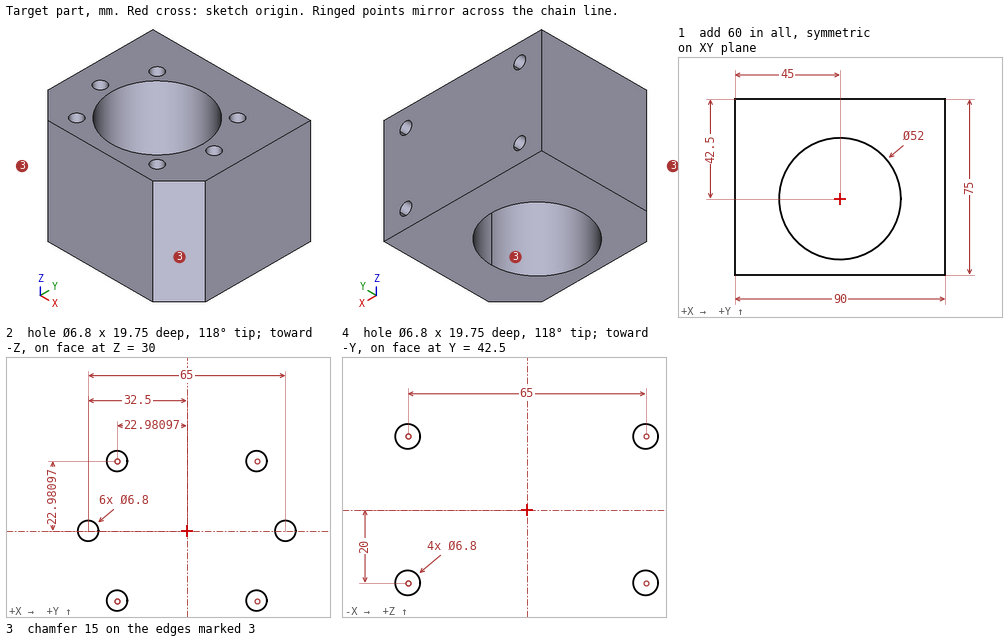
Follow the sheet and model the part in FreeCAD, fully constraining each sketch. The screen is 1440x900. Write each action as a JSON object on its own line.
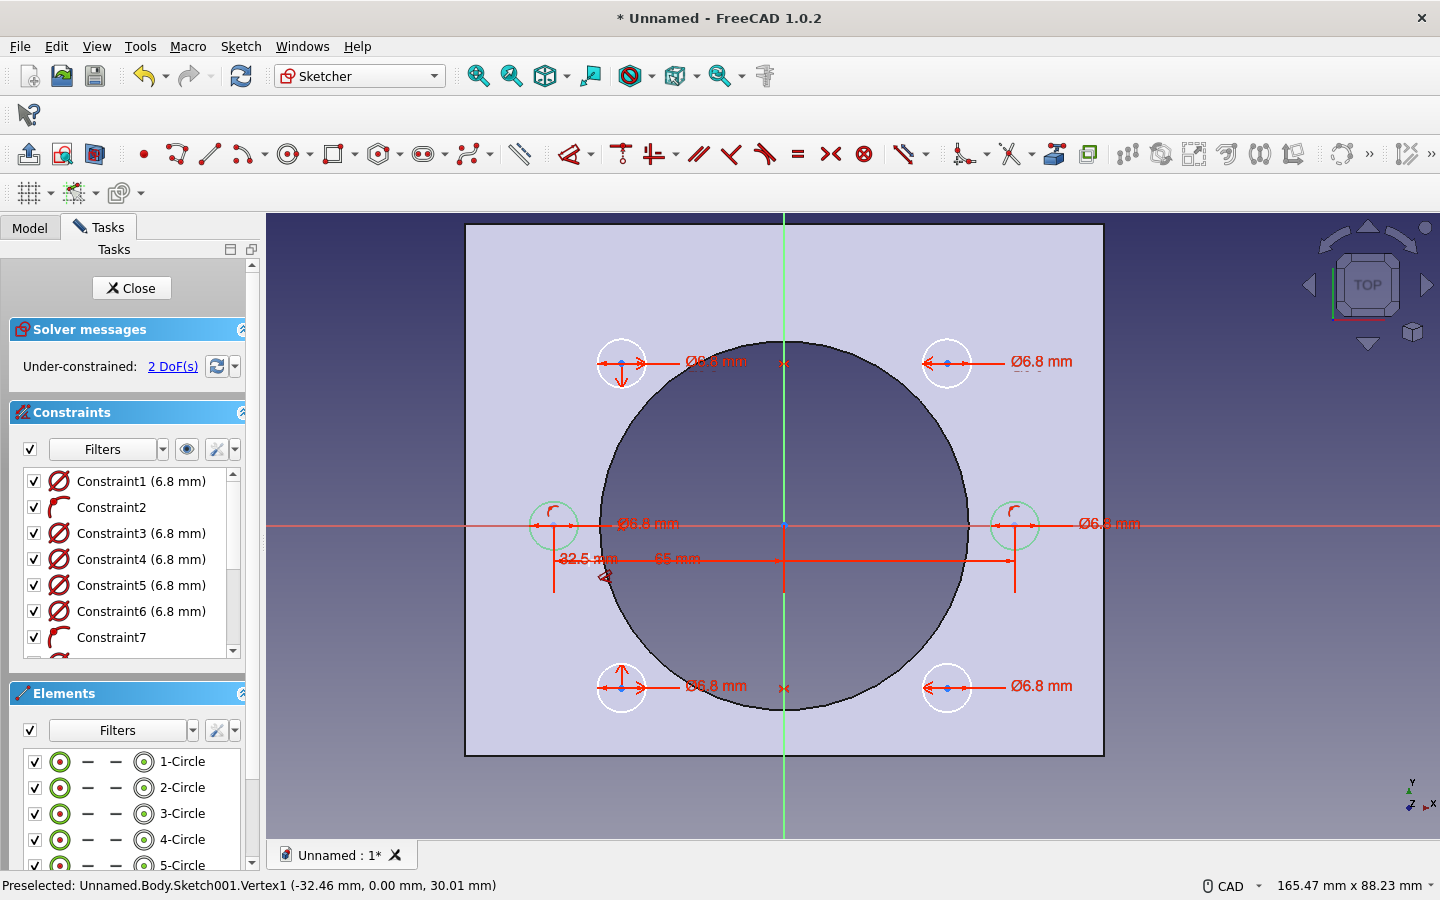
{"action": "left_click", "coordinate": [622, 363]}
{"action": "left_click", "coordinate": [703, 329]}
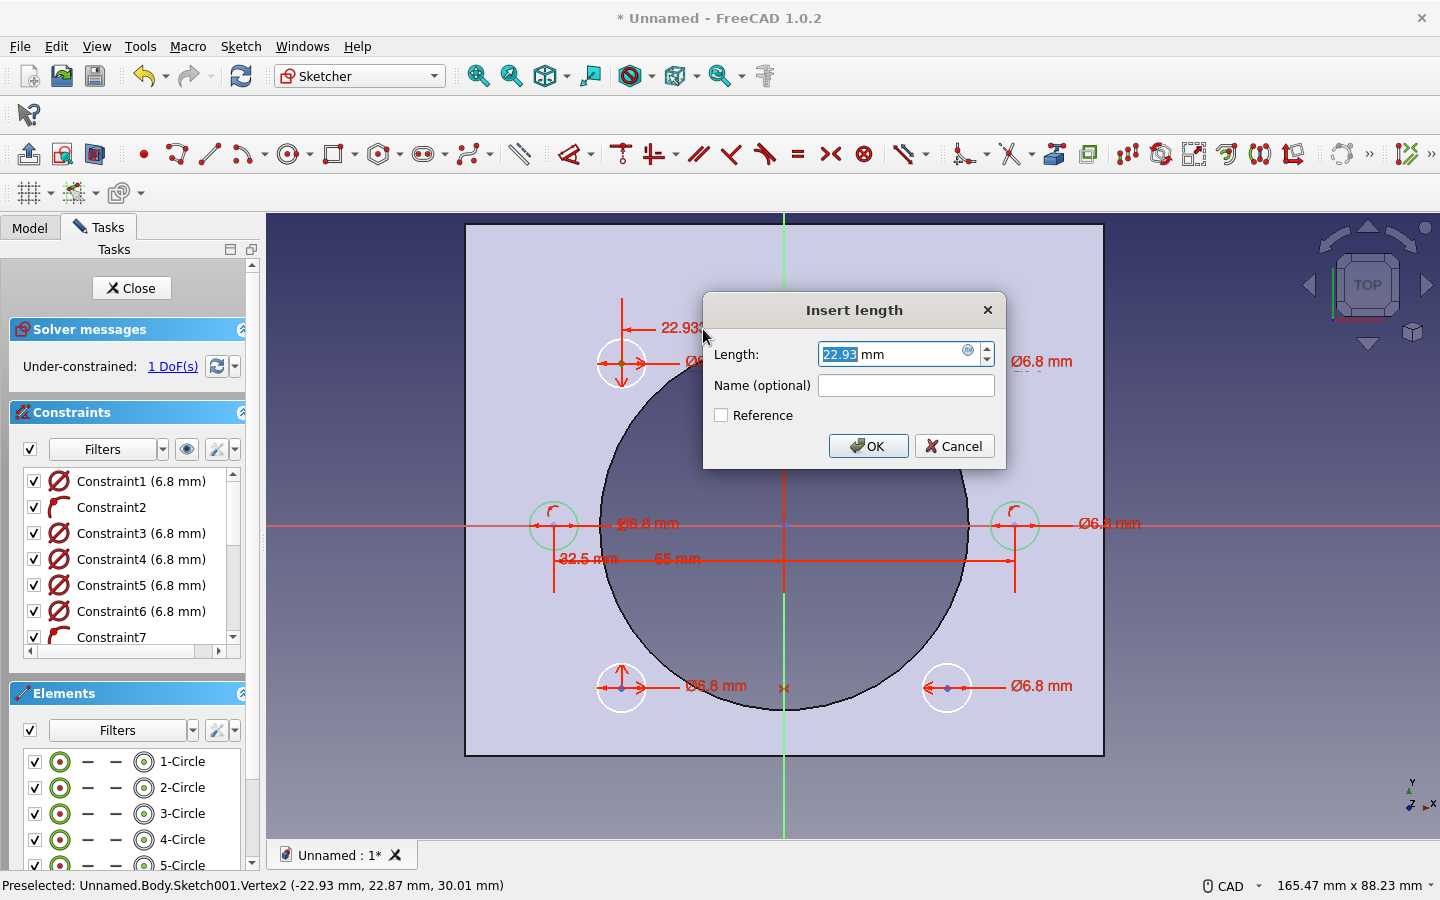
{"action": "type", "text": "22.98097"}
{"action": "key", "text": "Return"}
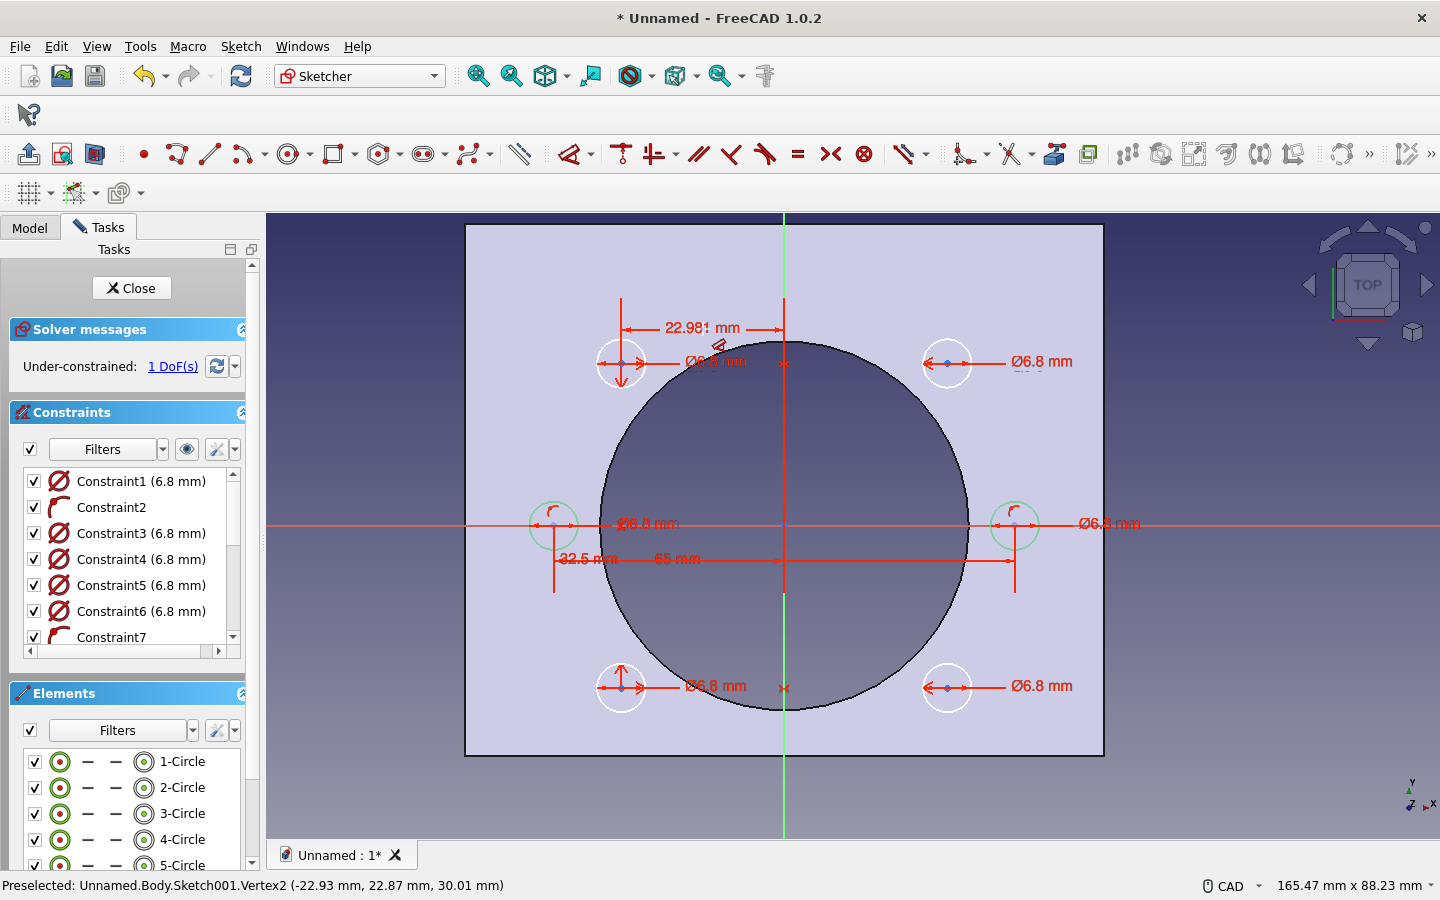
{"action": "left_click", "coordinate": [621, 363]}
{"action": "left_click", "coordinate": [587, 445]}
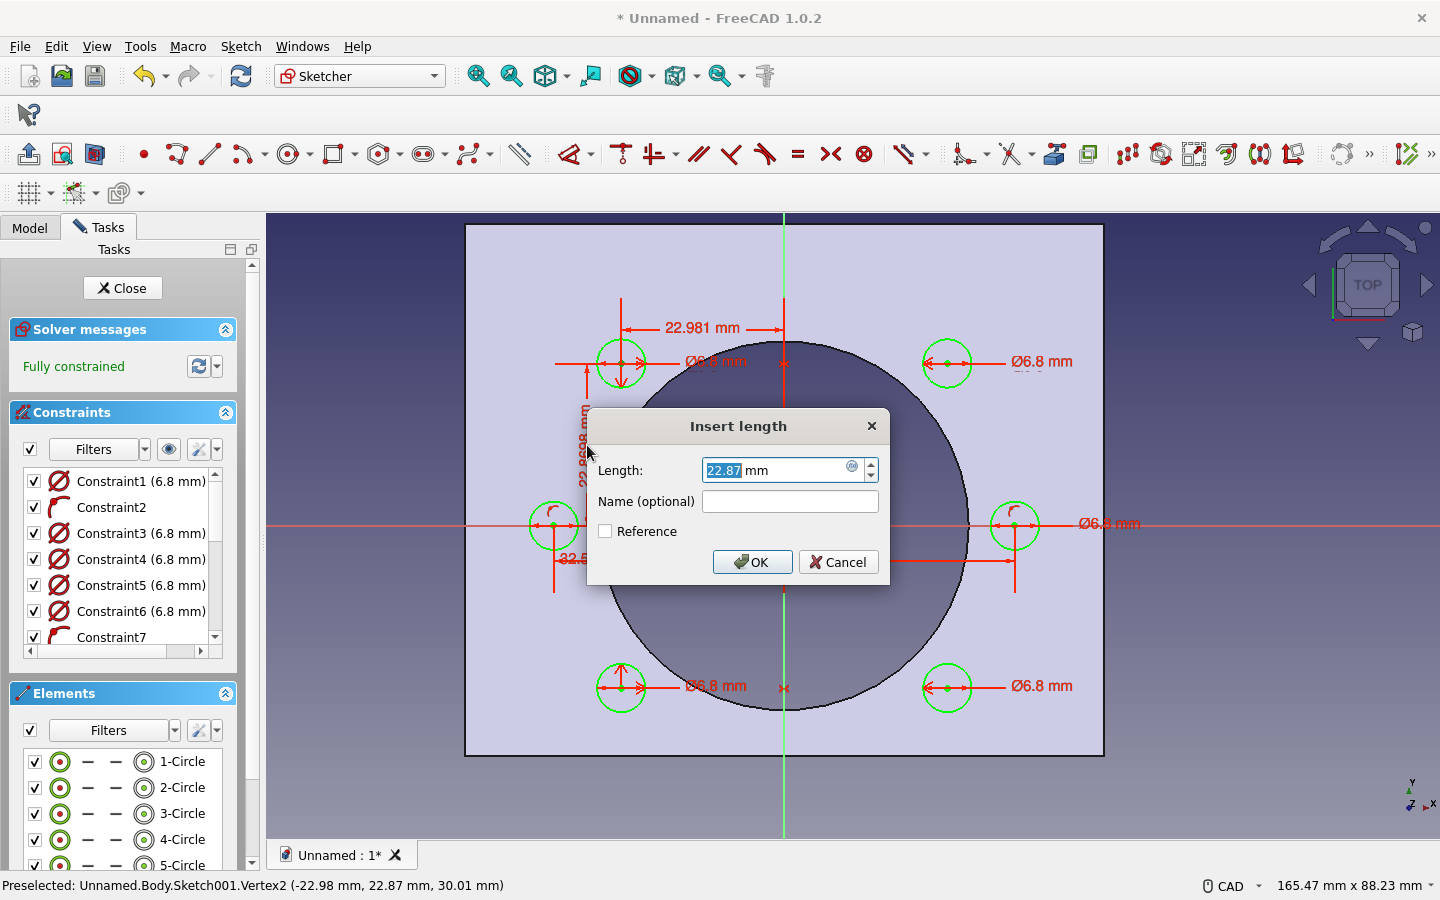
{"action": "type", "text": "22.98097"}
{"action": "key", "text": "Return"}
{"action": "key", "text": "Escape"}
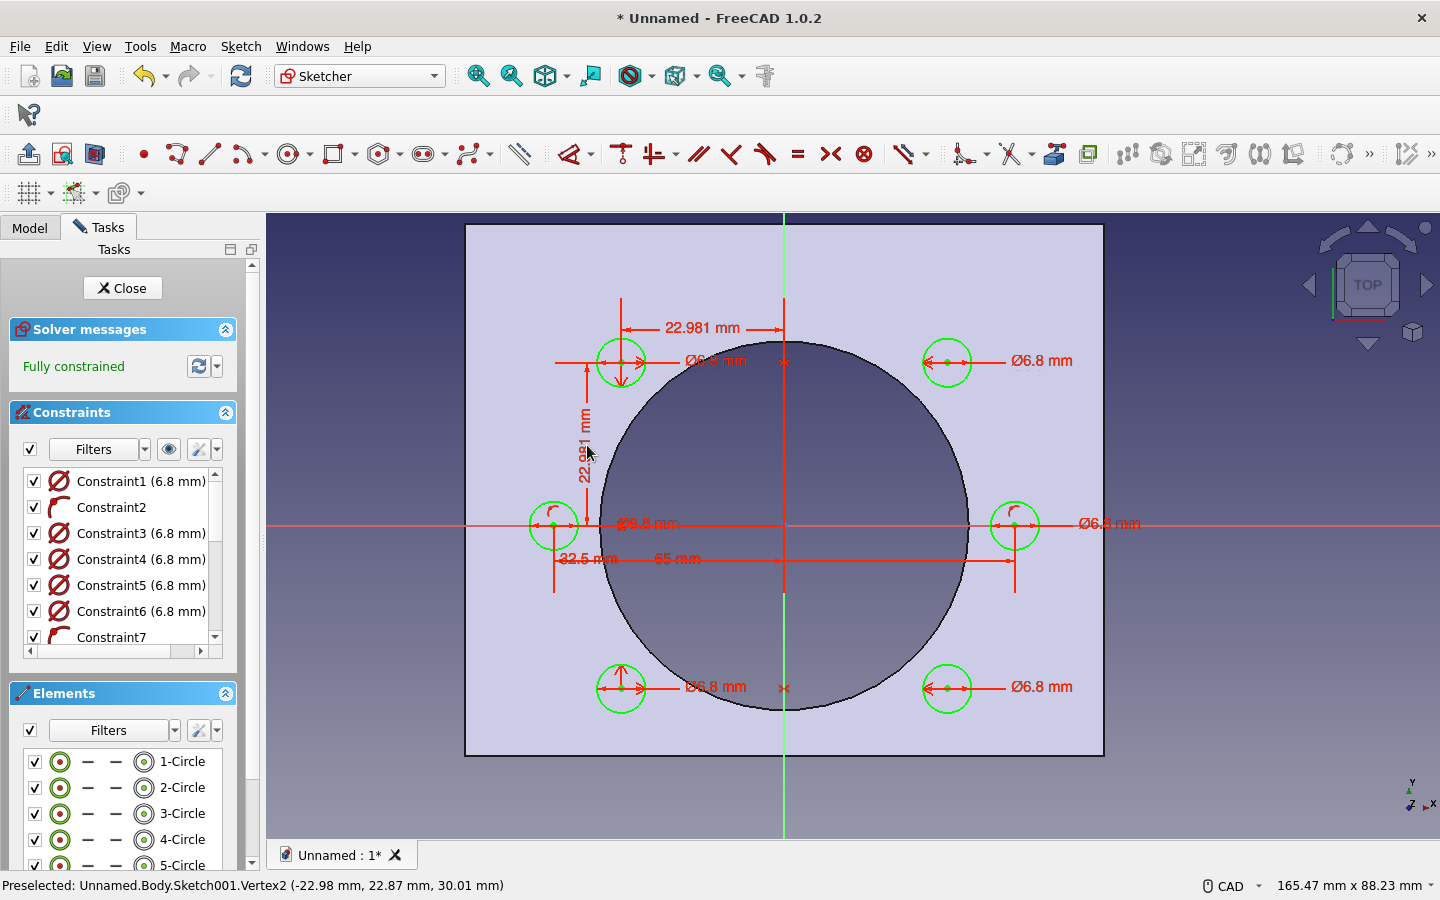
{"action": "left_click", "coordinate": [123, 288]}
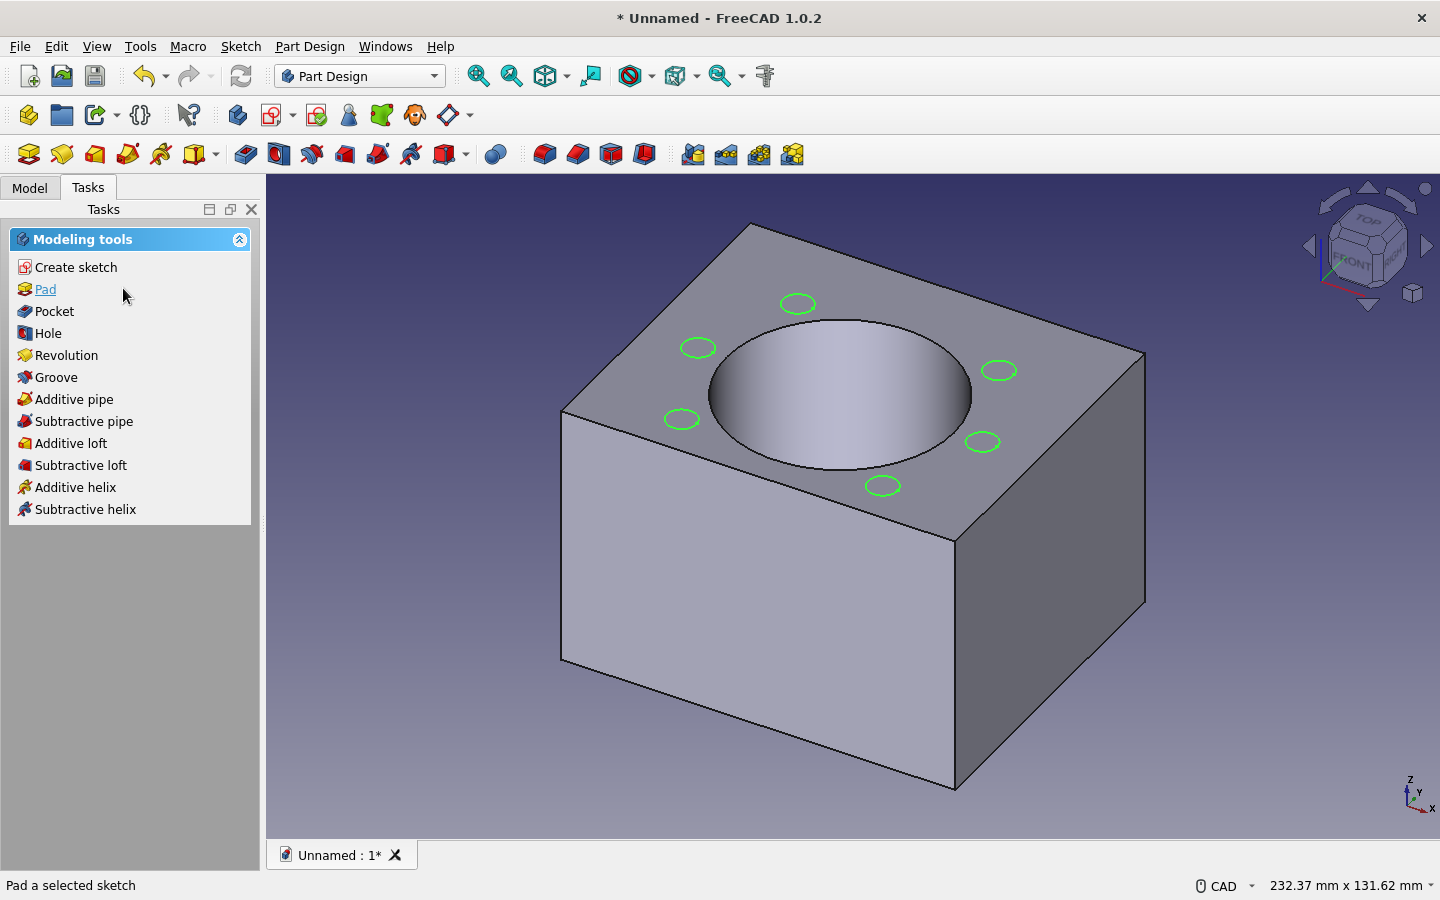
{"action": "left_click", "coordinate": [279, 154]}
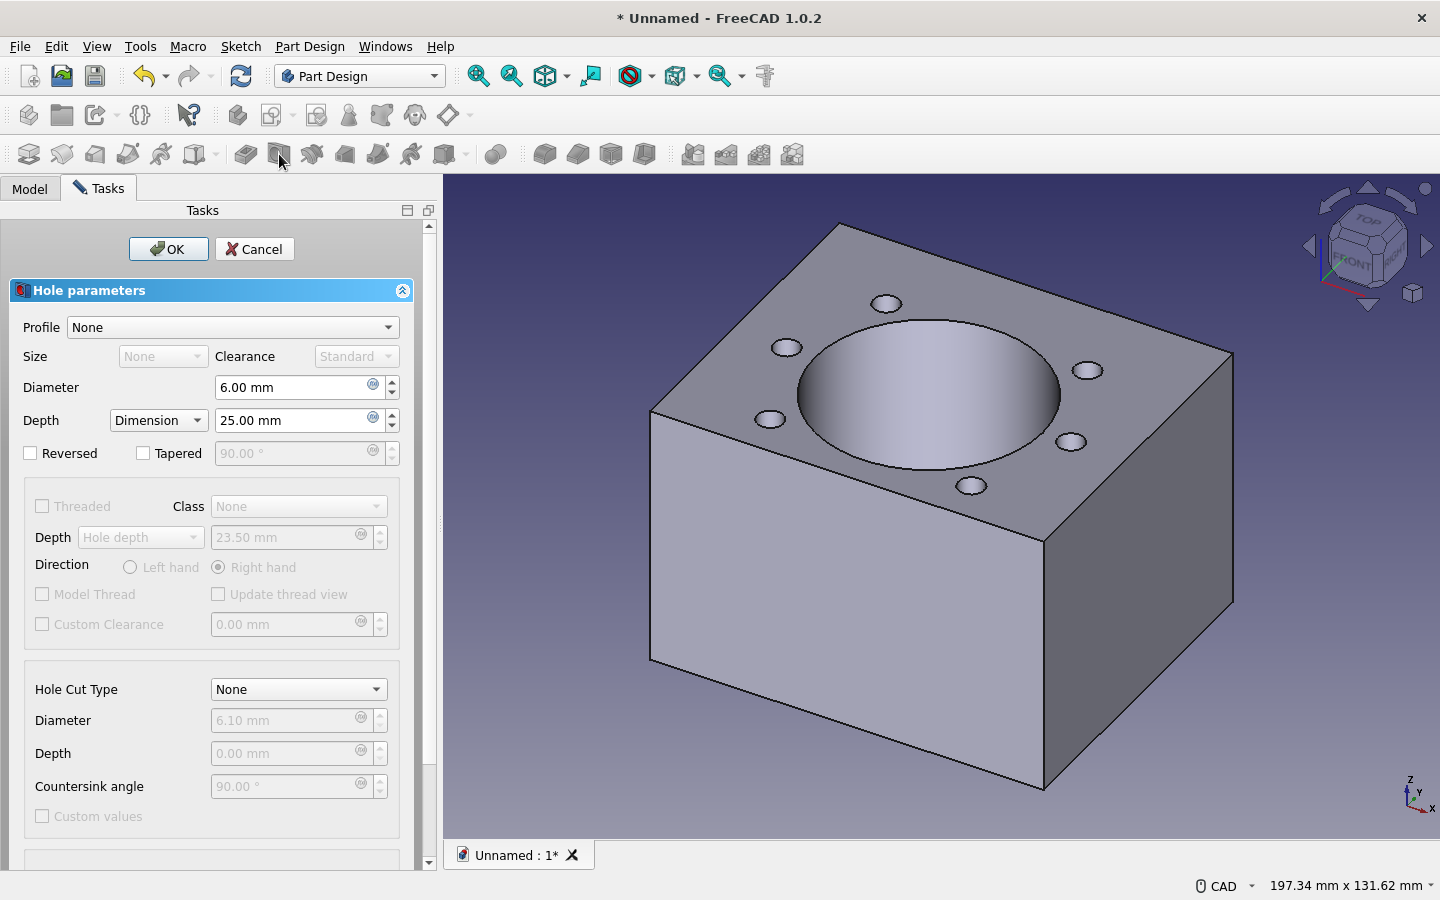
{"action": "triple_click", "coordinate": [300, 388]}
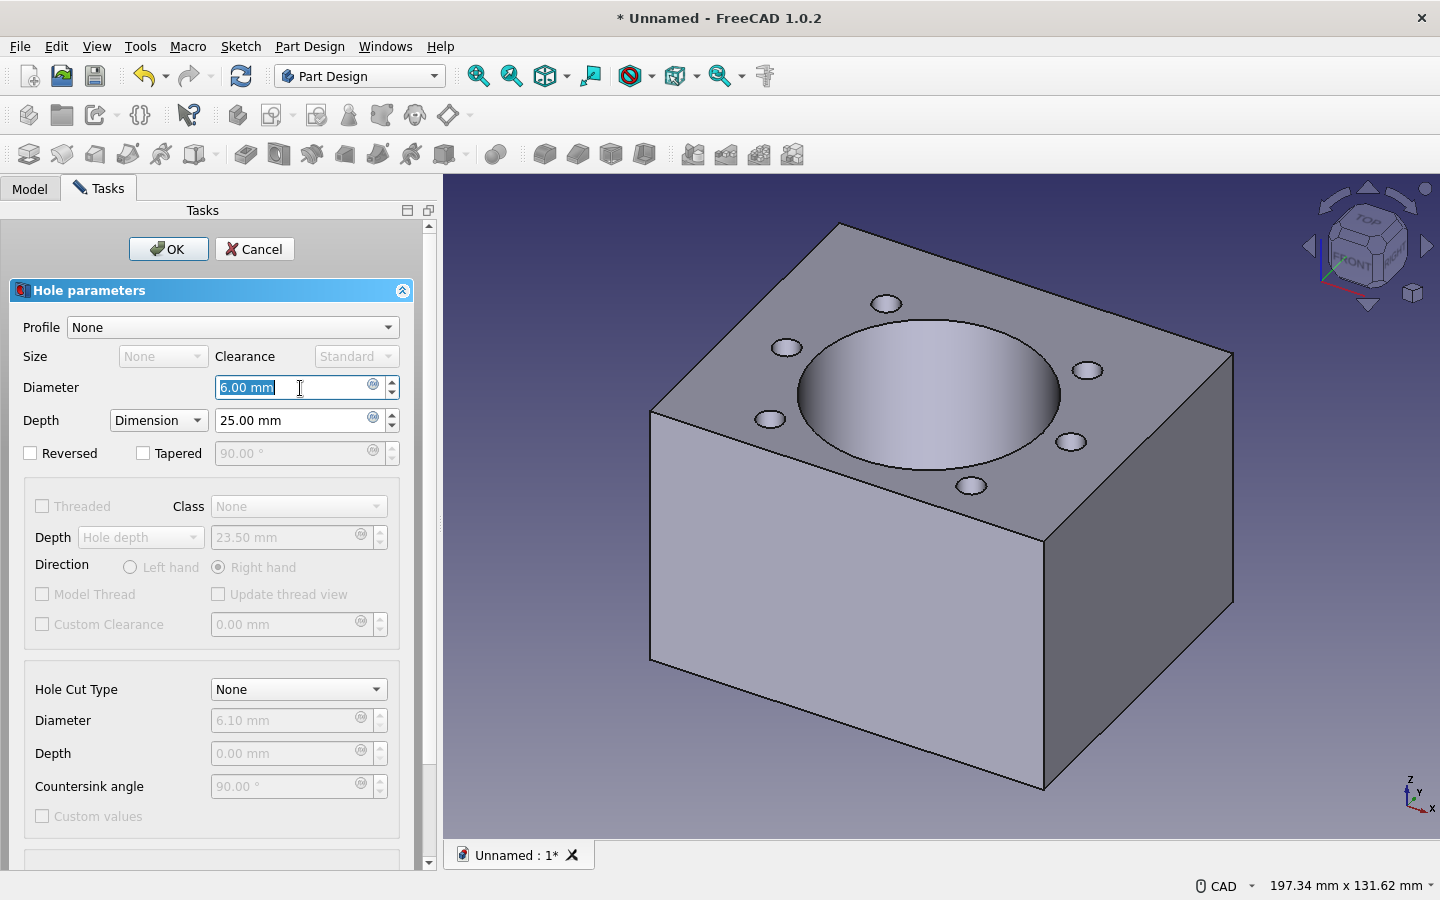
{"action": "type", "text": "6.8"}
{"action": "key", "text": "Tab"}